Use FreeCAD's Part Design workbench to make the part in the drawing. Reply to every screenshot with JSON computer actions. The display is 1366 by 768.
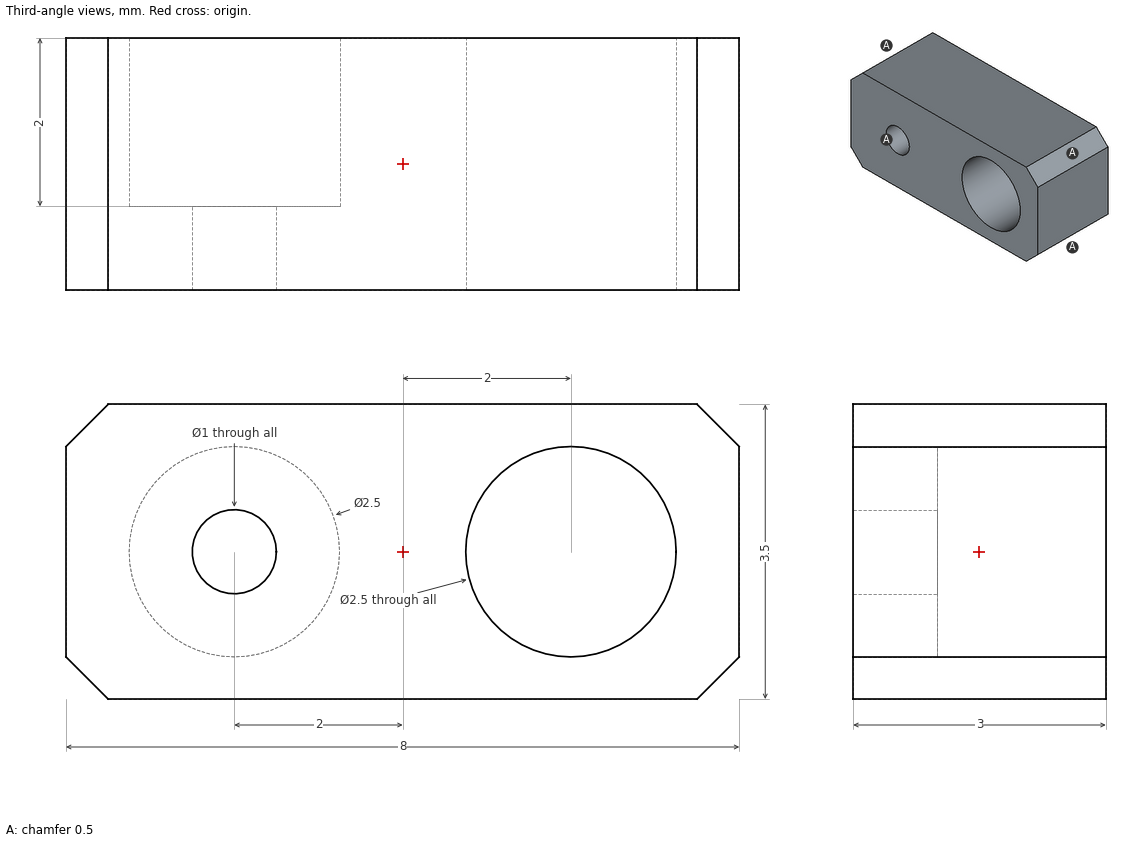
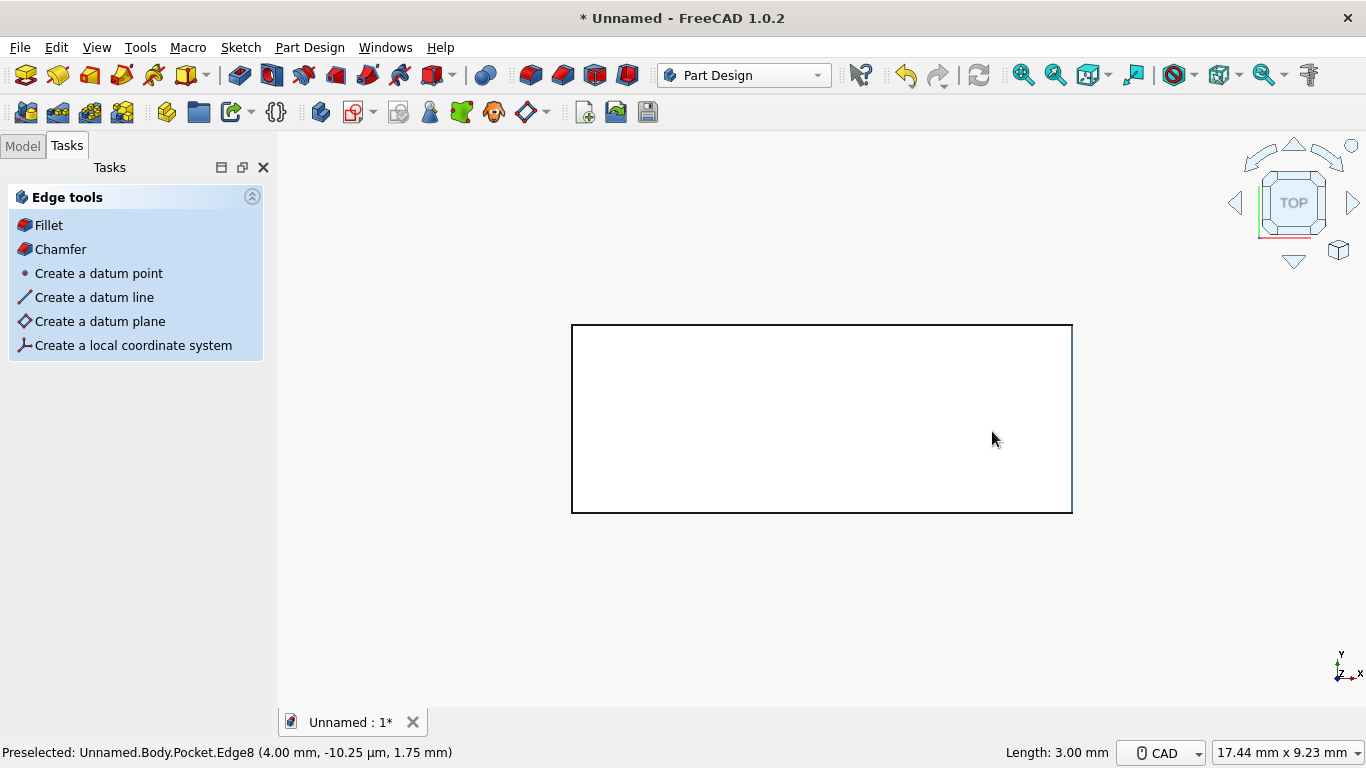
{"action": "left_click", "coordinate": [572, 418], "text": "ctrl"}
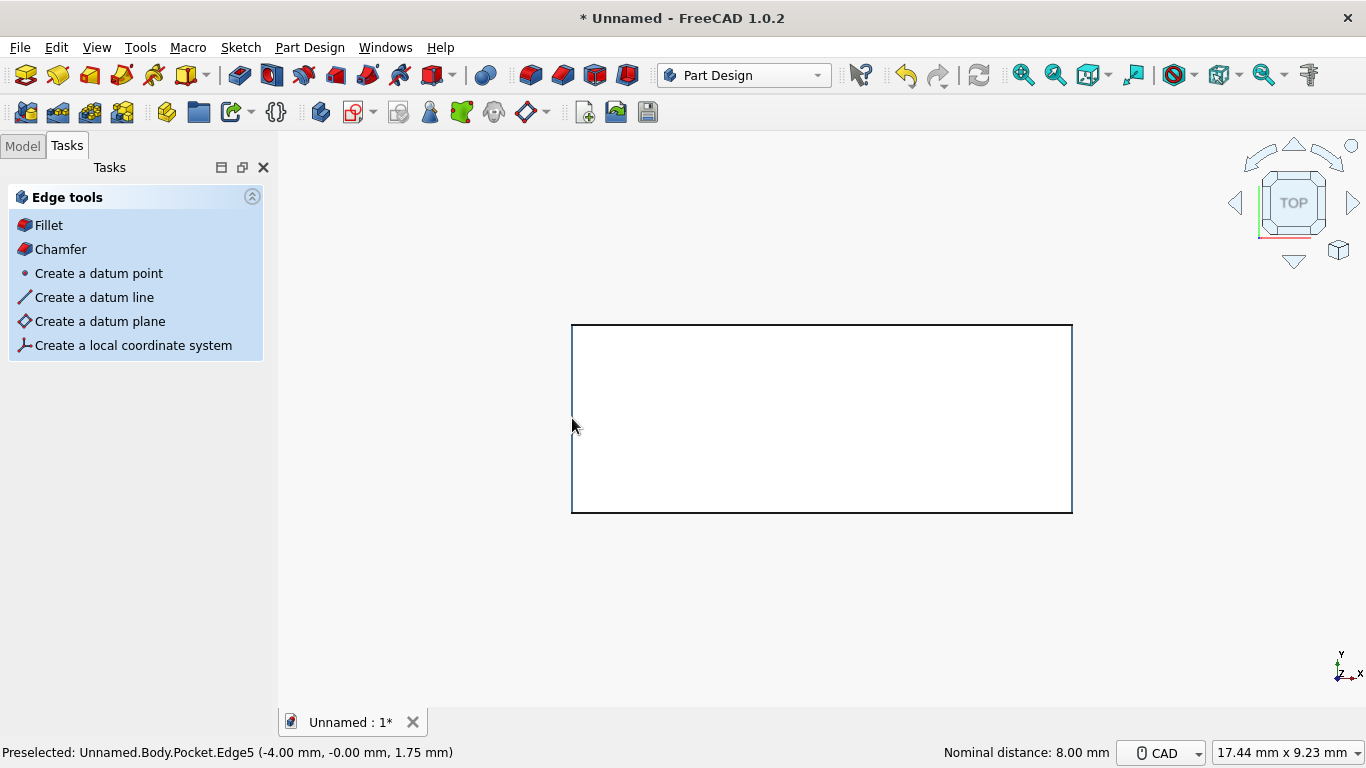
{"action": "key", "text": "1"}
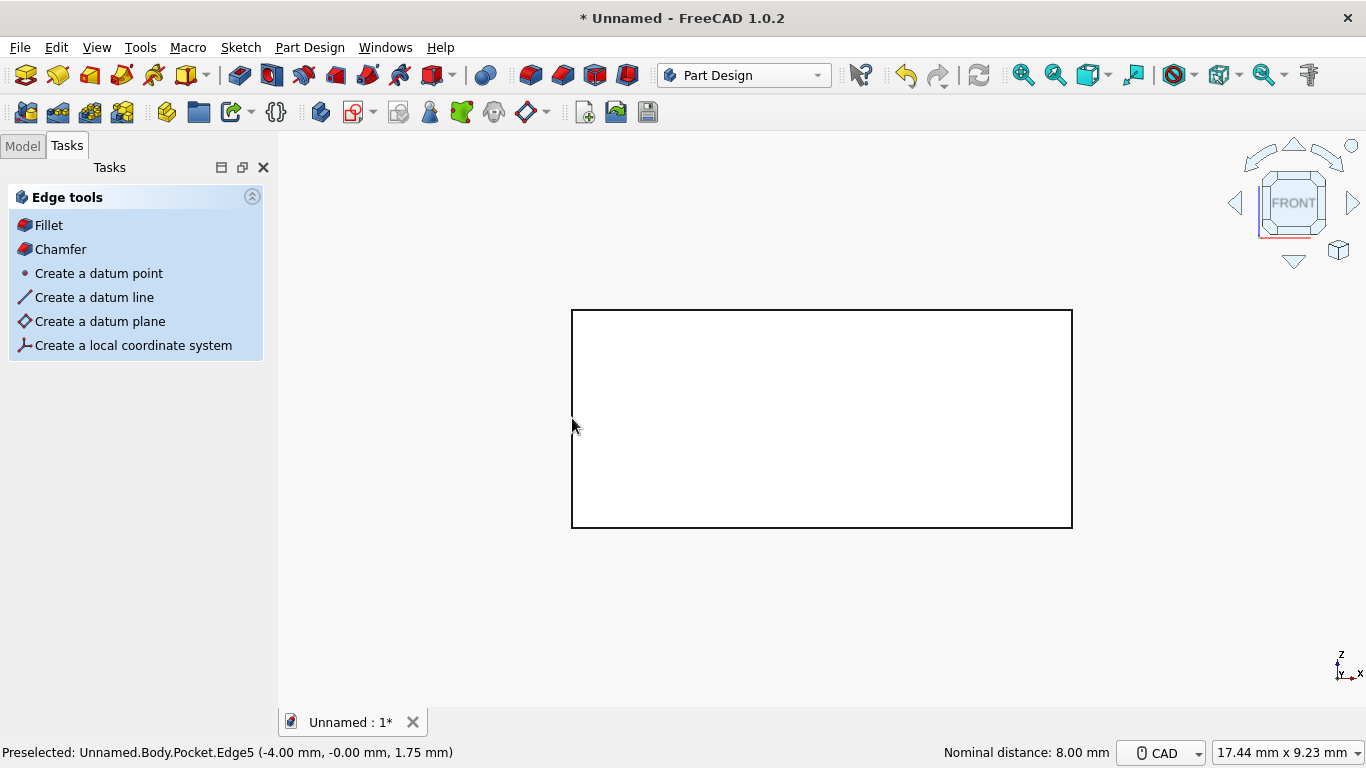
{"action": "key", "text": "3"}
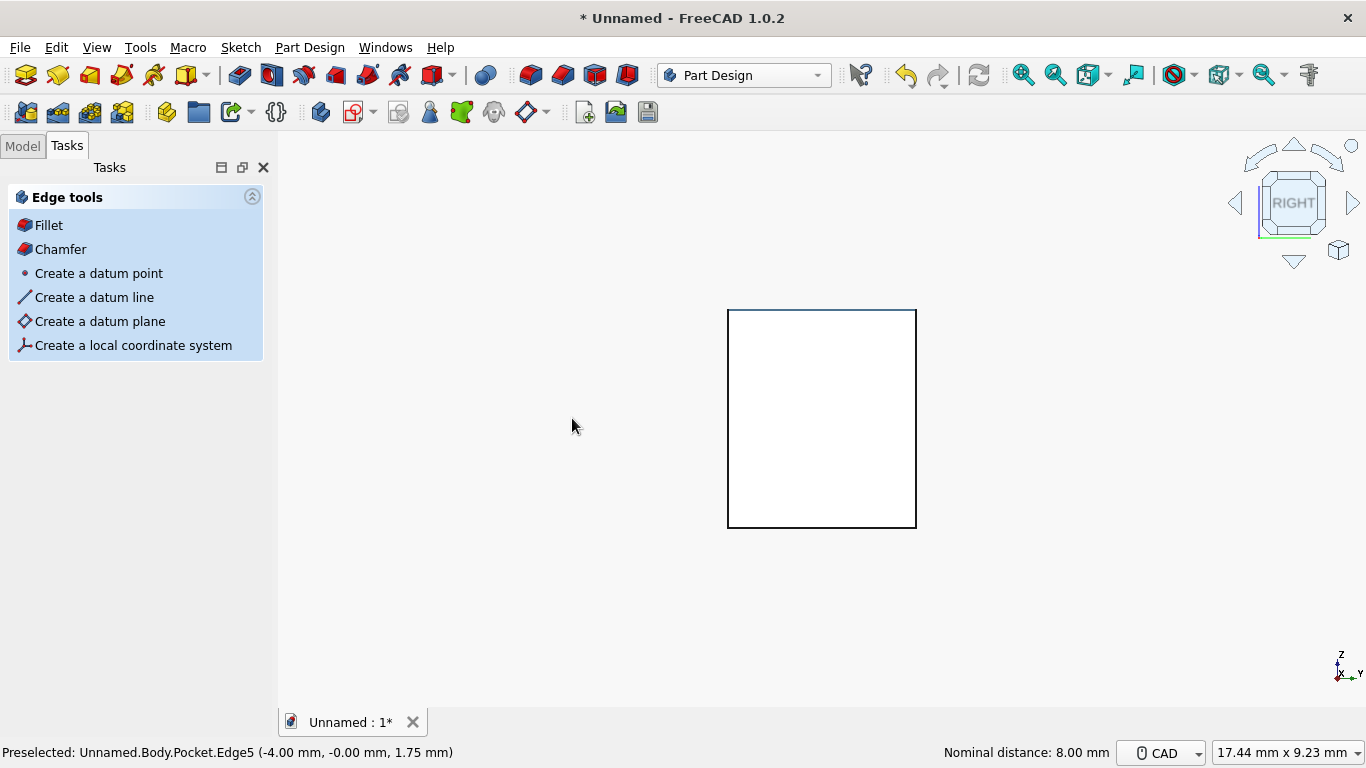
{"action": "left_click", "coordinate": [1024, 76]}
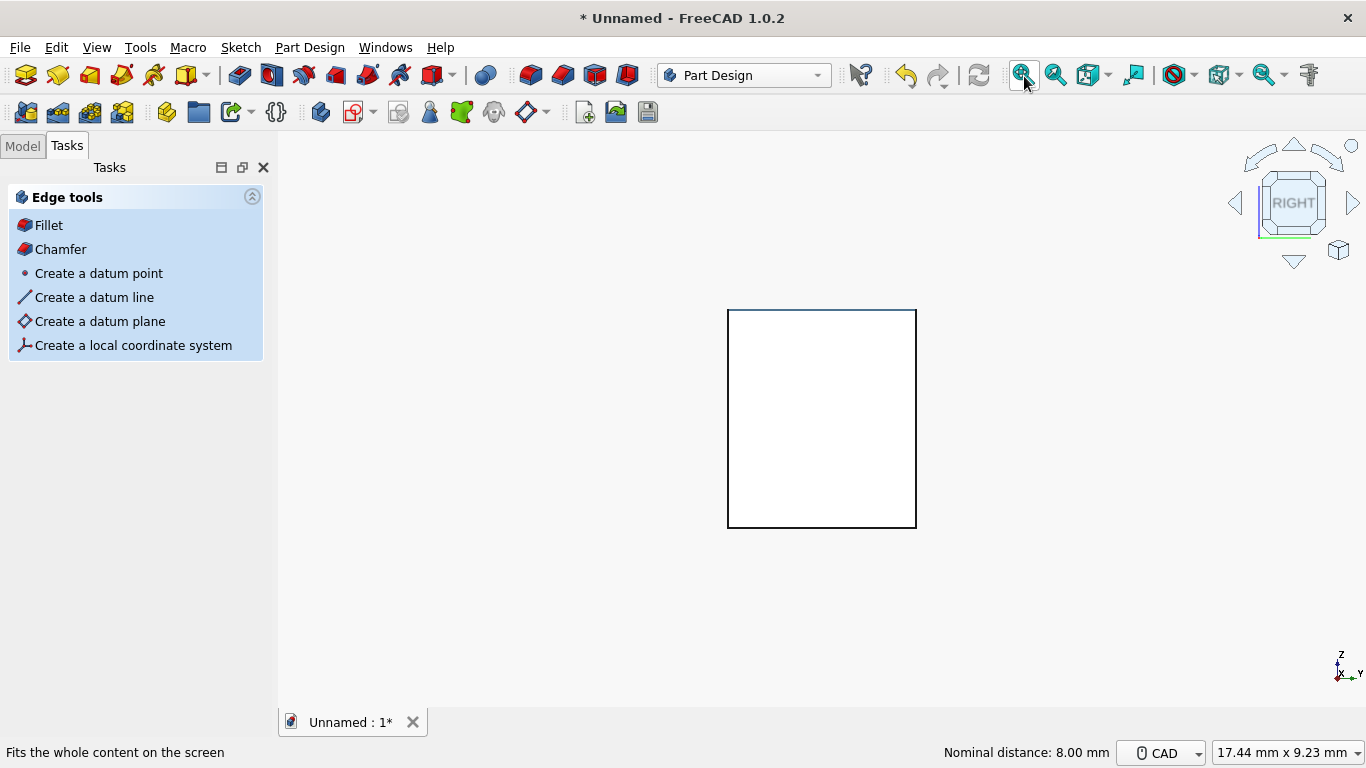
{"action": "left_click", "coordinate": [822, 527], "text": "ctrl"}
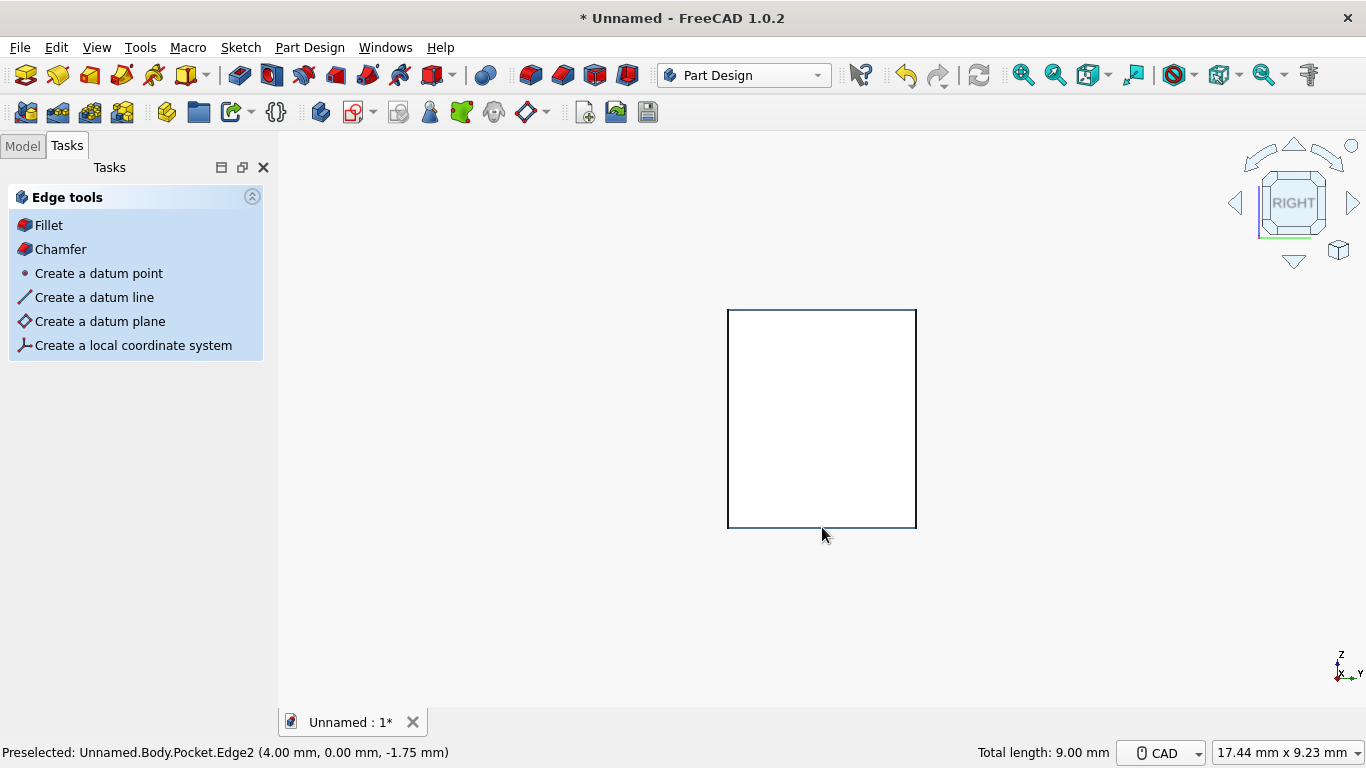
{"action": "key", "text": "5"}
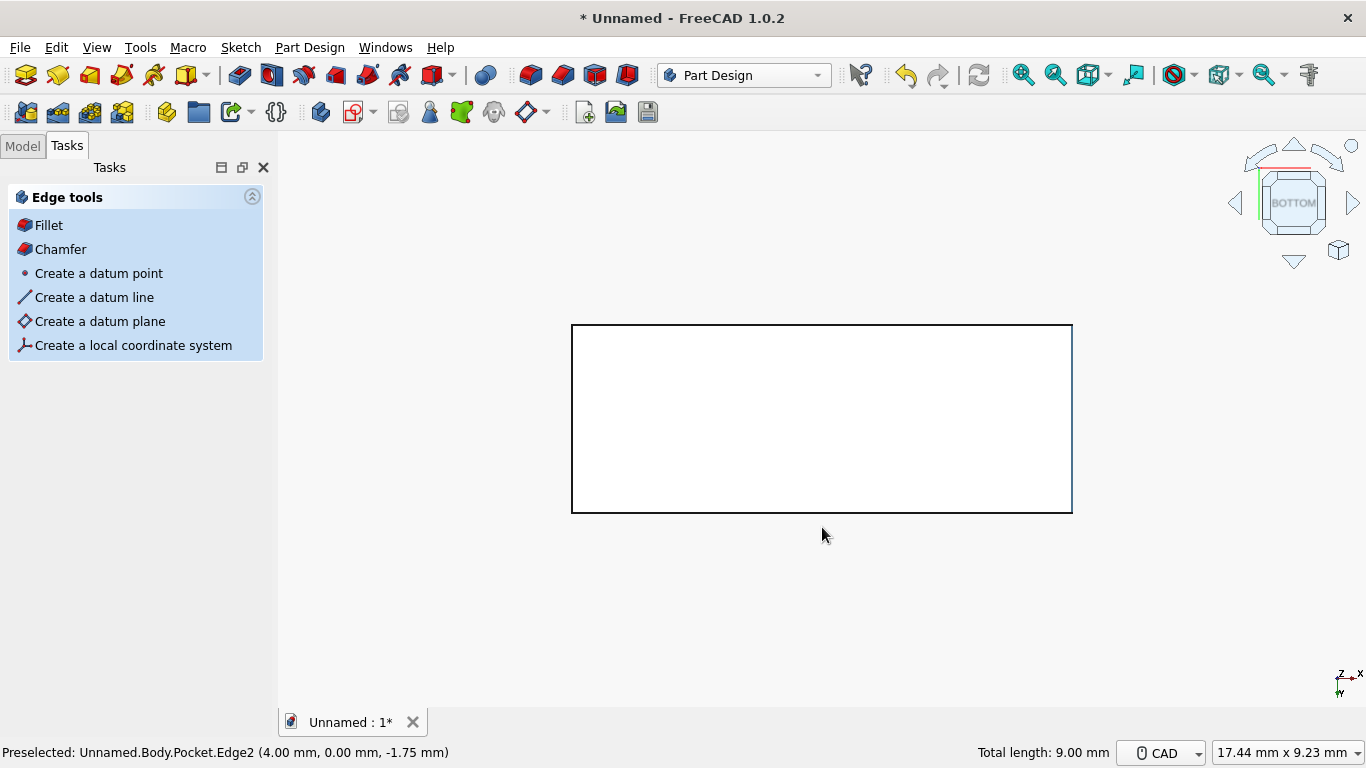
{"action": "left_click", "coordinate": [572, 418], "text": "ctrl"}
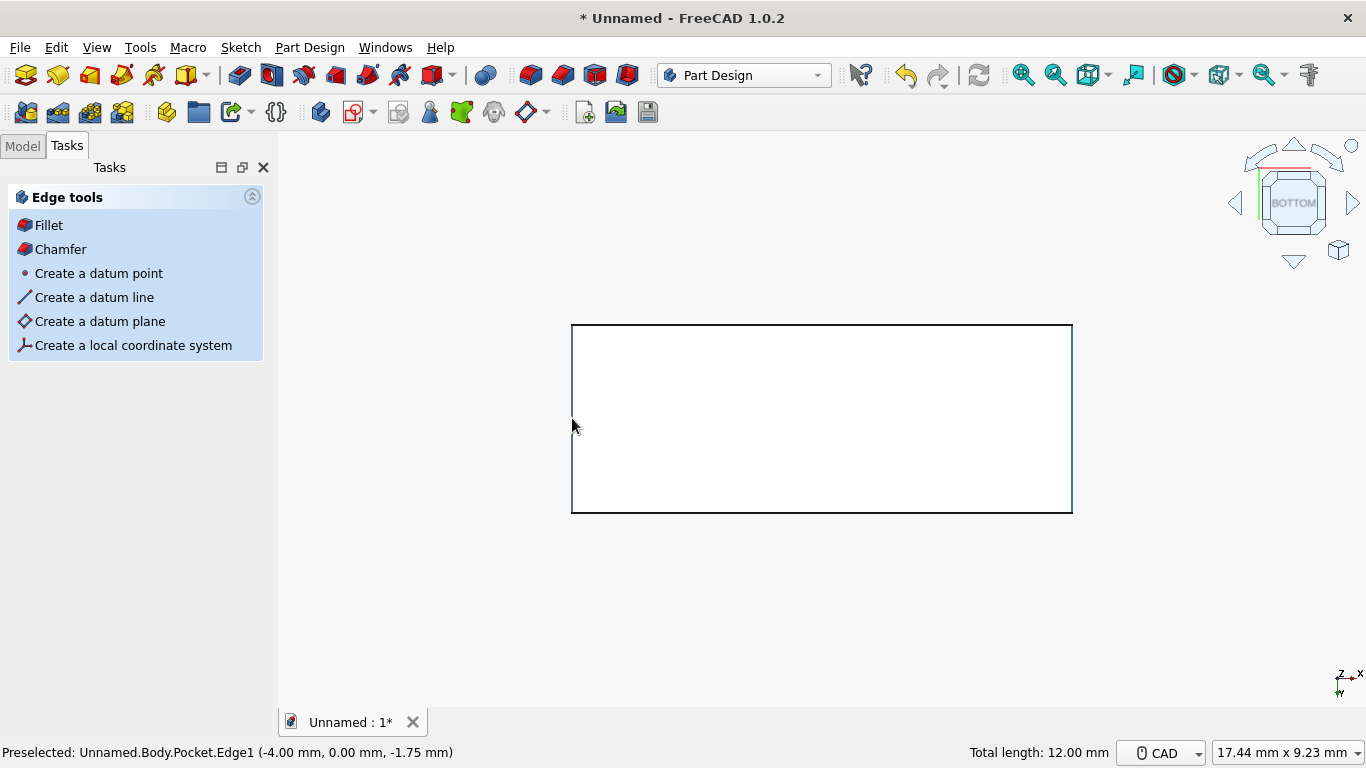
{"action": "left_click", "coordinate": [564, 76]}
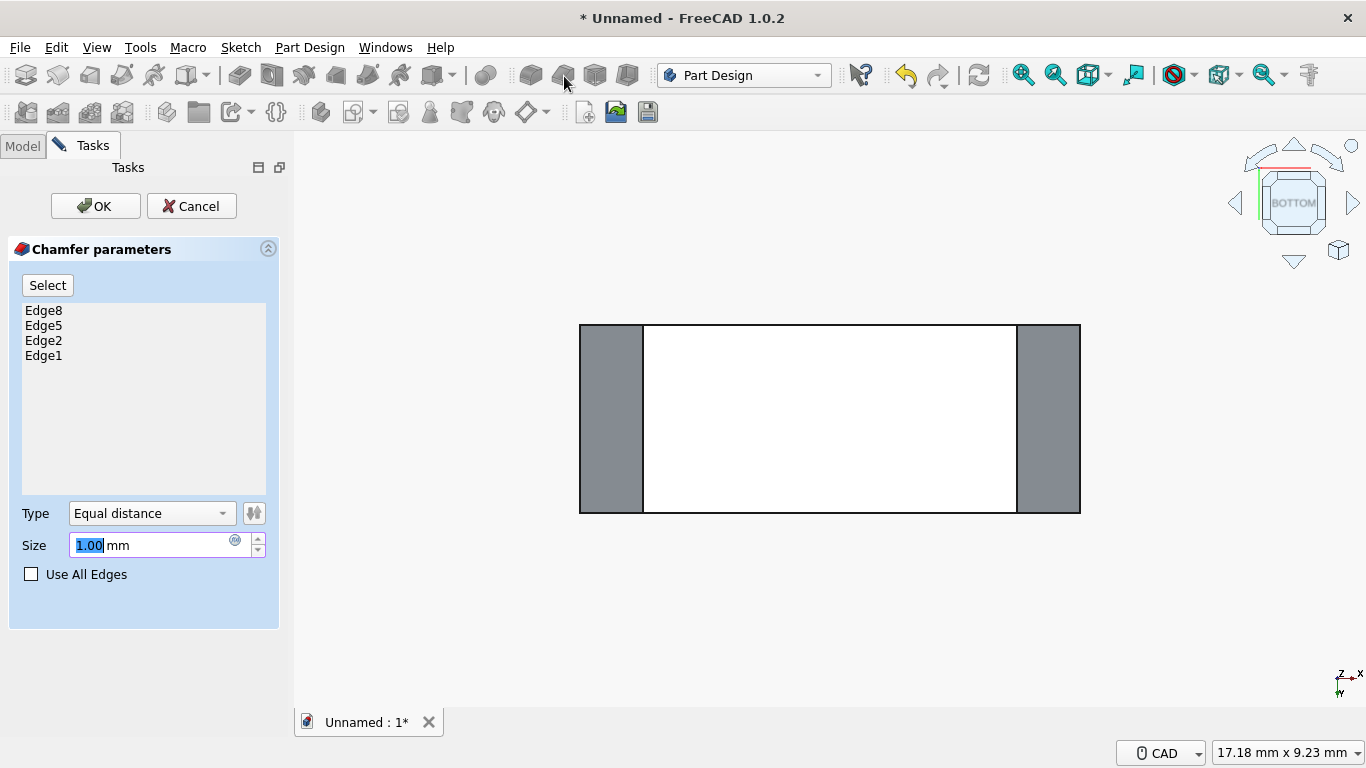
{"action": "type", "text": "0.5"}
{"action": "key", "text": "Tab"}